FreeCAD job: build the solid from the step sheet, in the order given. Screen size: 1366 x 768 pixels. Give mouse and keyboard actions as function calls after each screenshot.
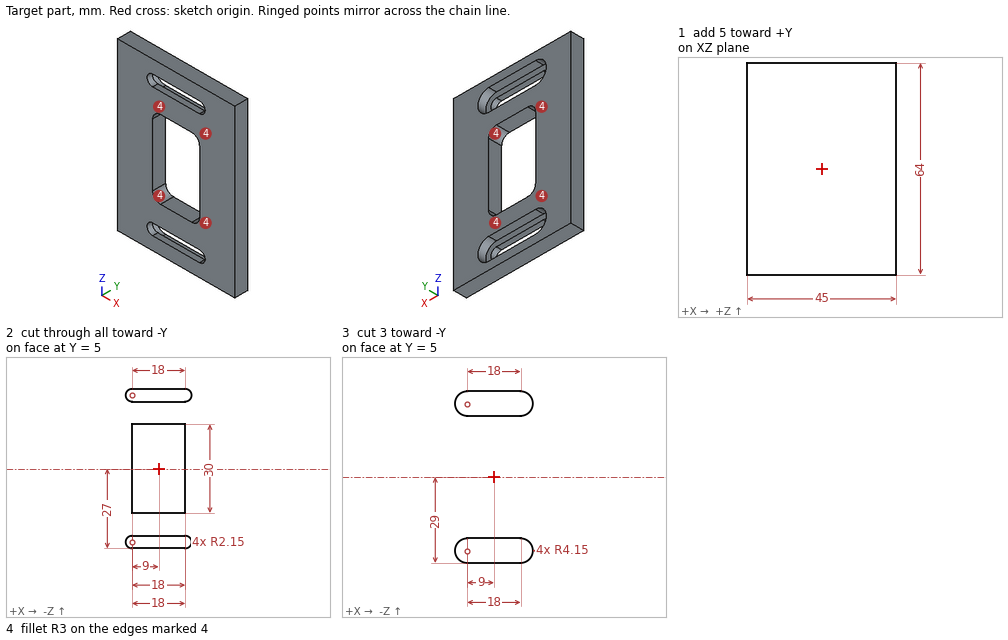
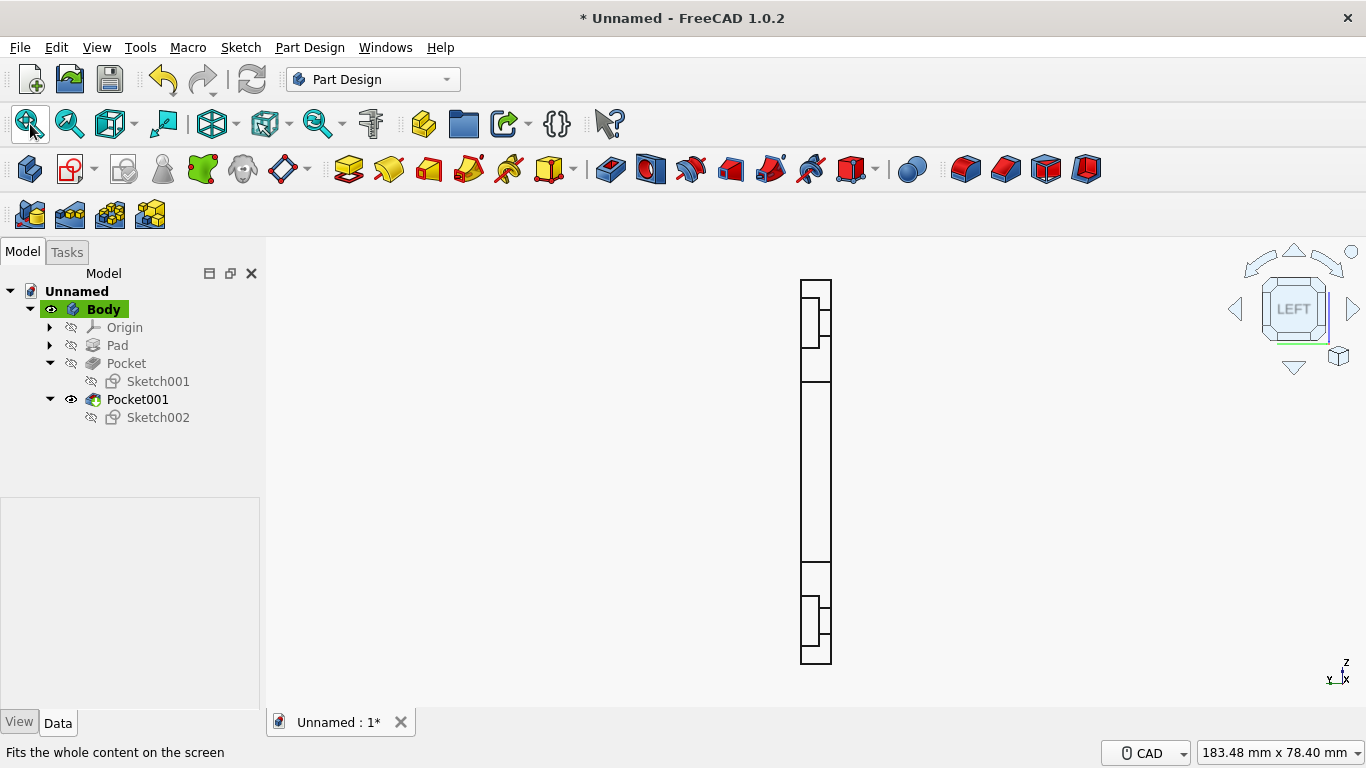
key(0)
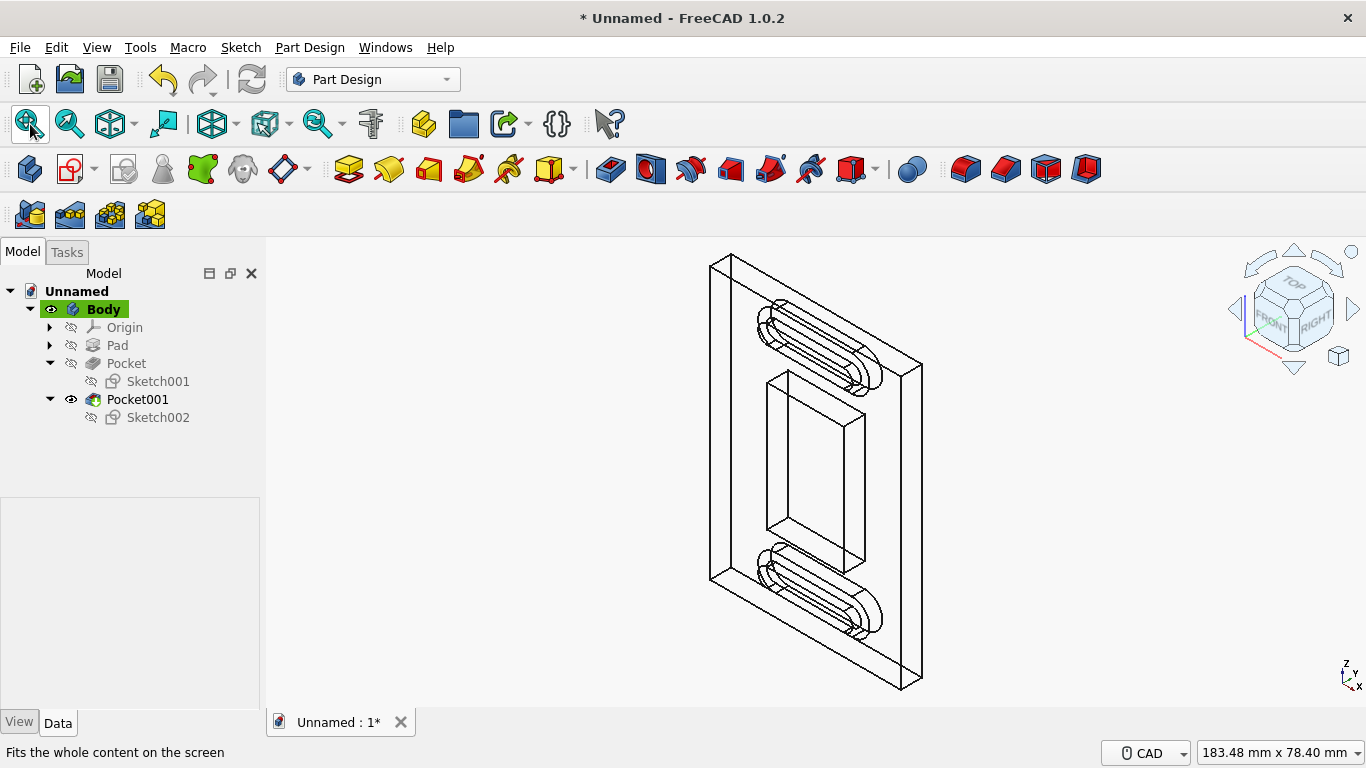
click(778, 522)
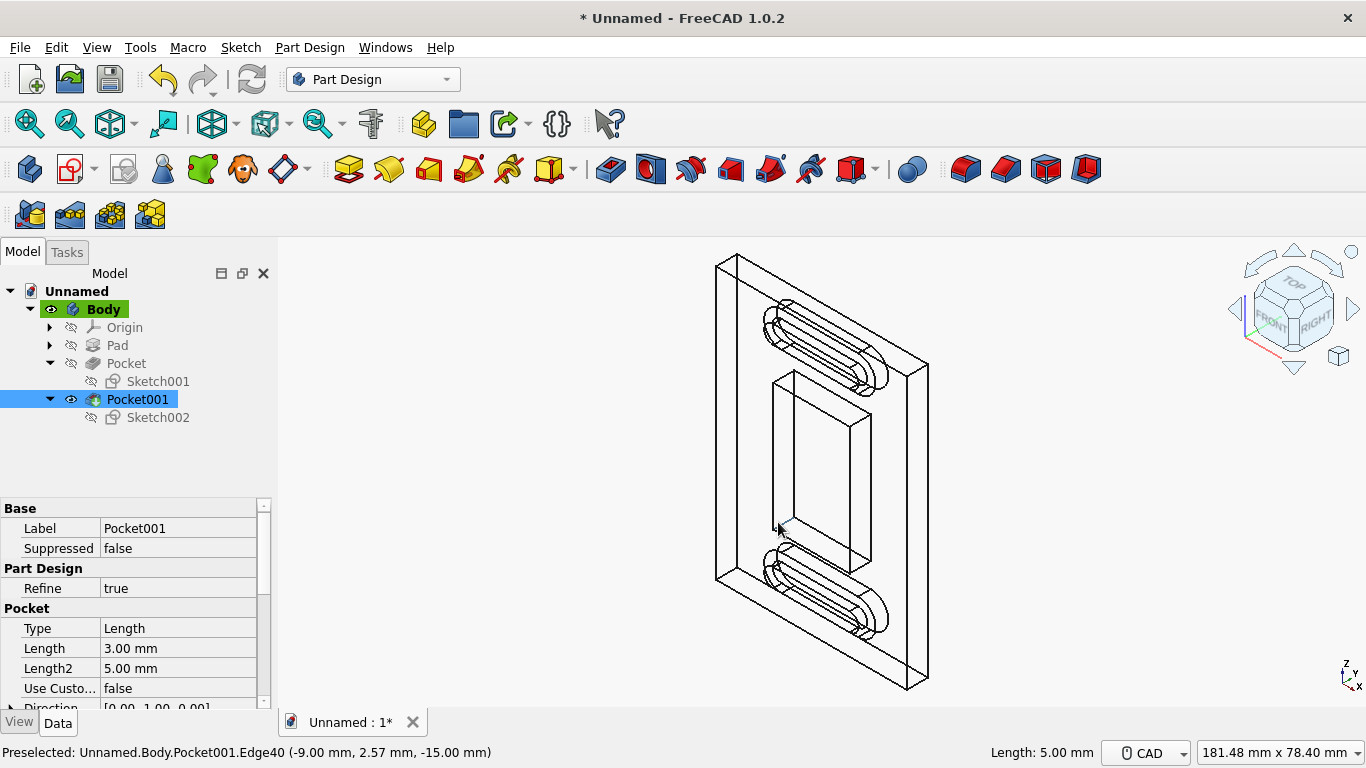
click(860, 566, ctrl)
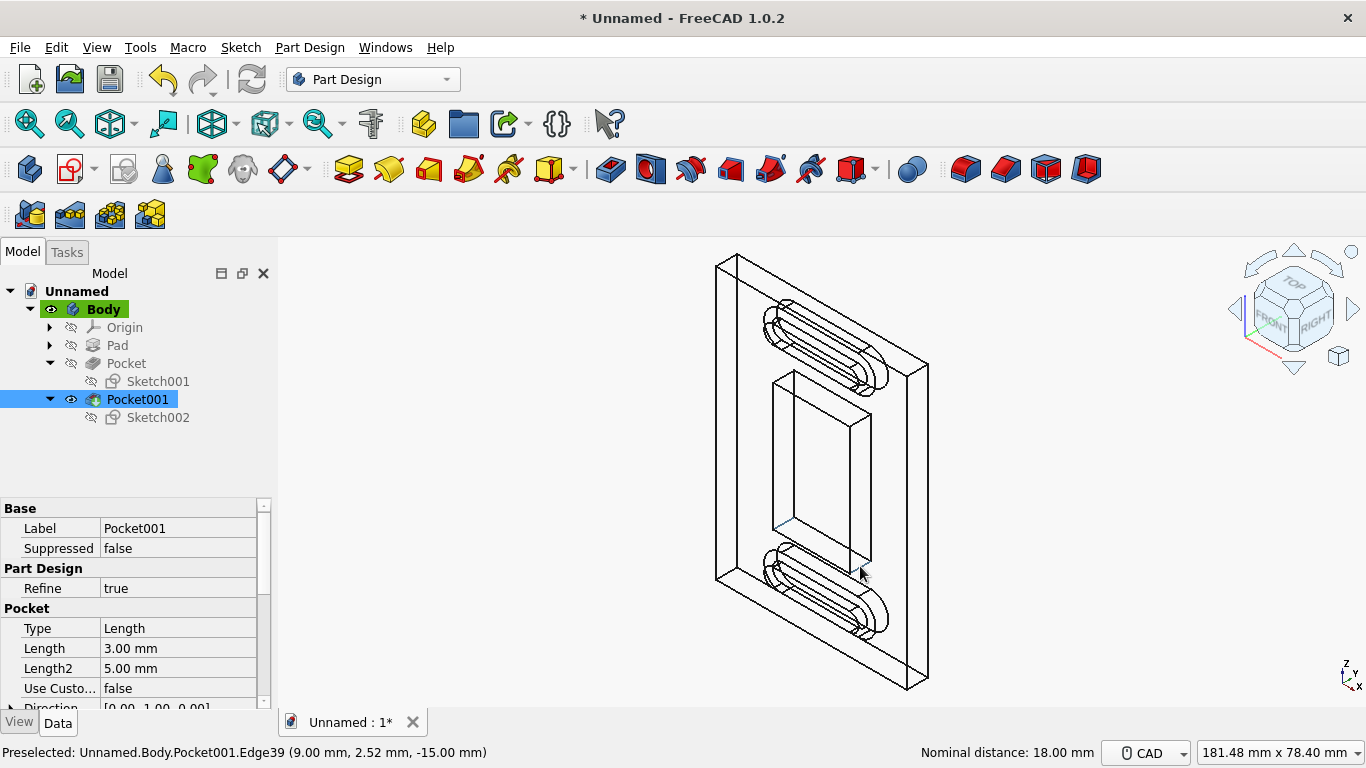
click(860, 420, ctrl)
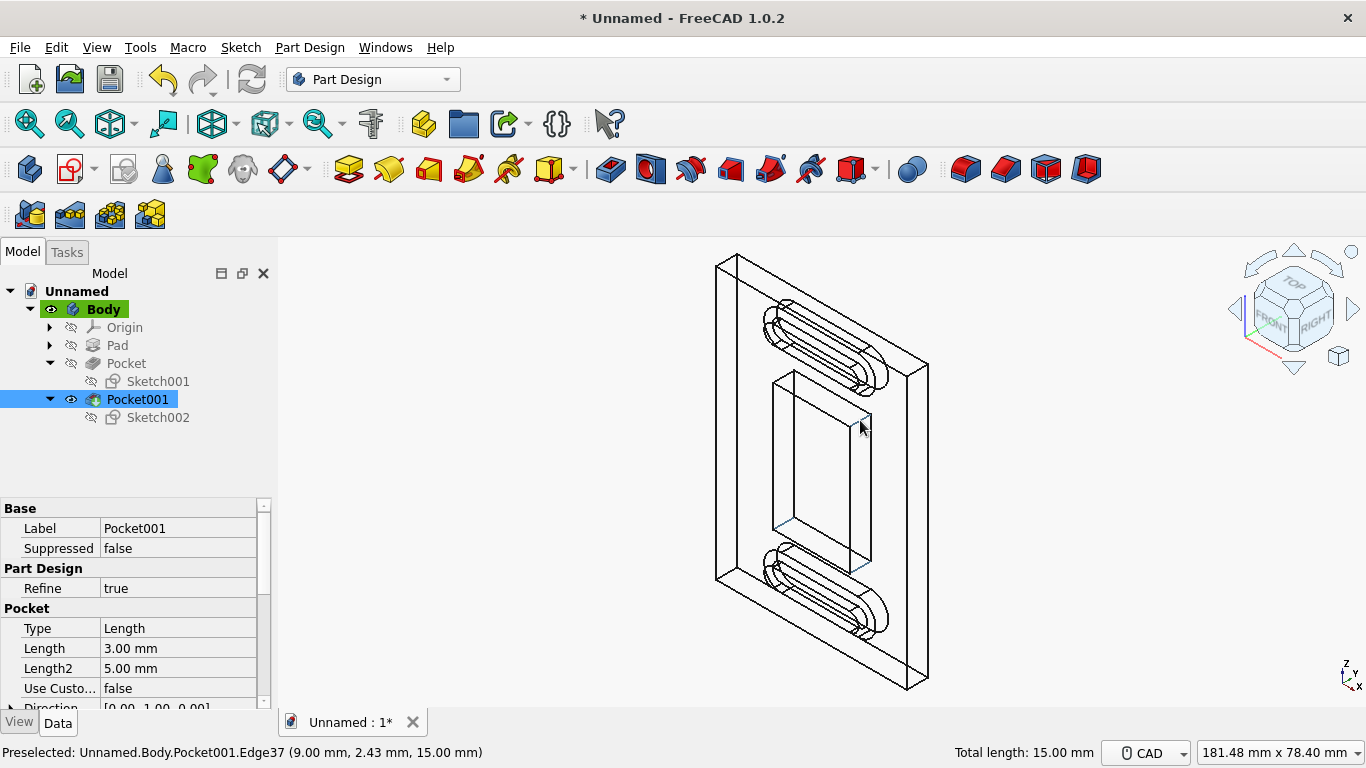
click(784, 376, ctrl)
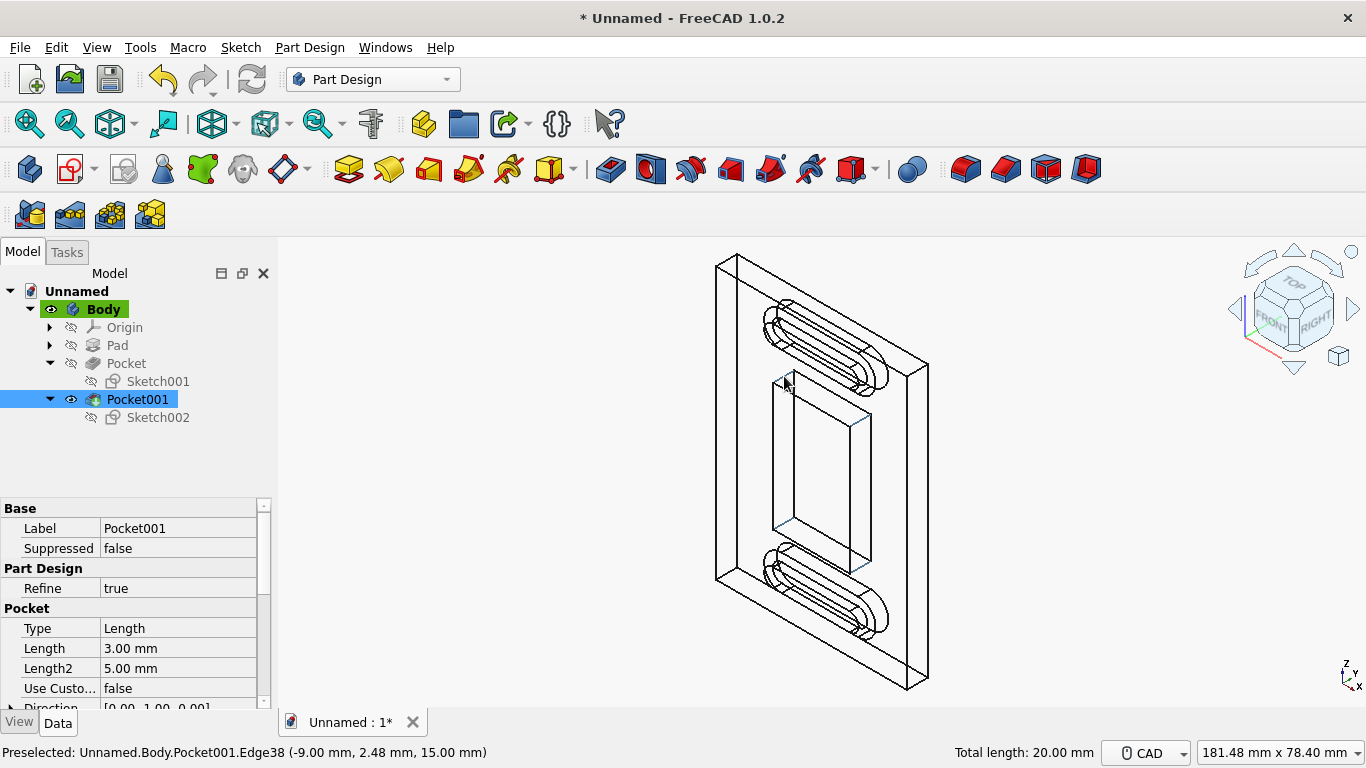
key(v)
key(1)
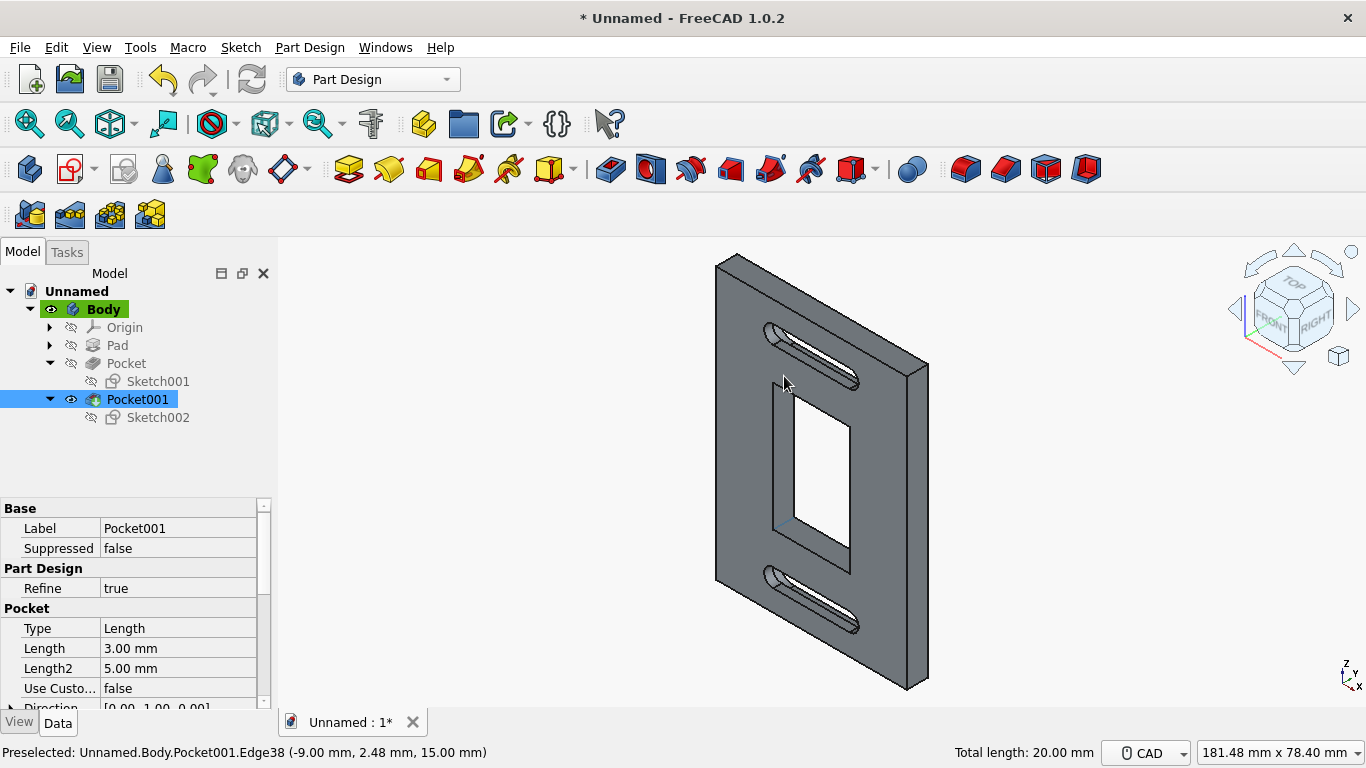
click(966, 170)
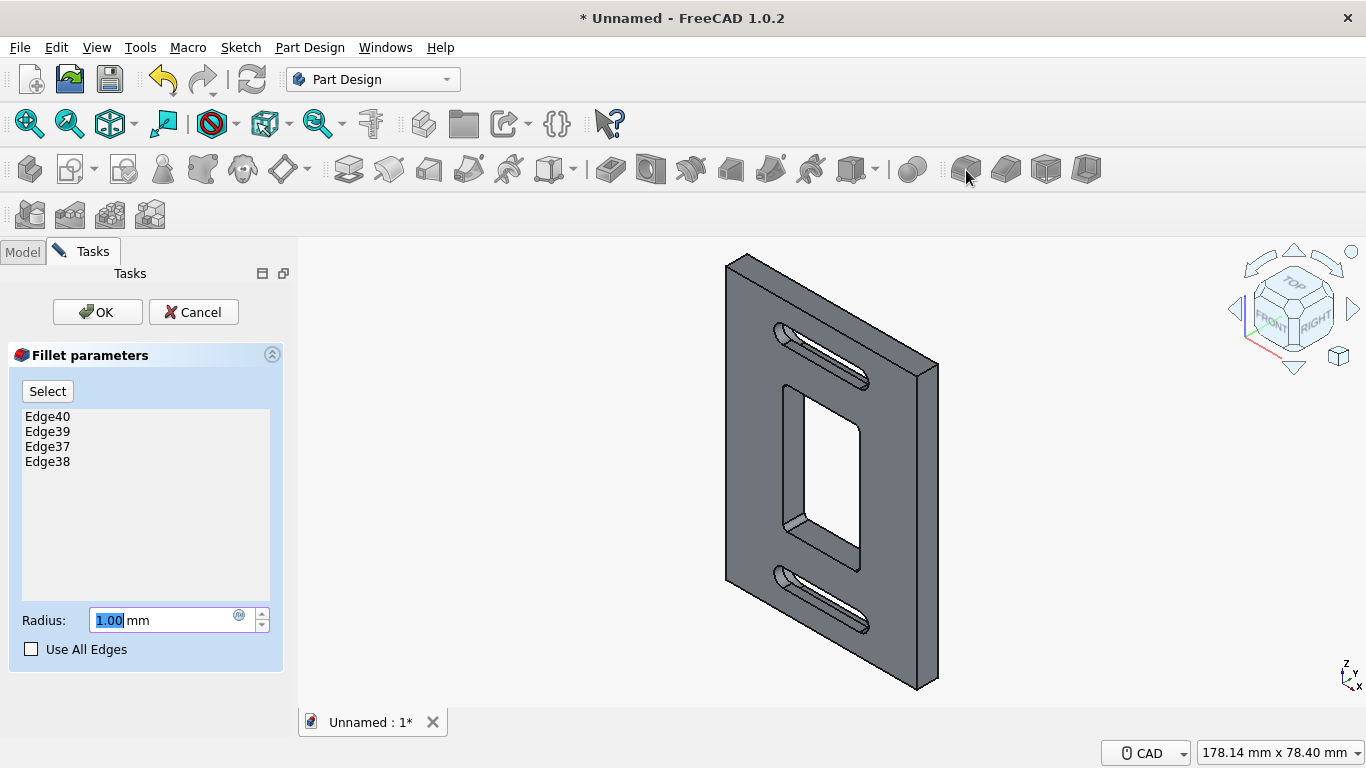
text(3)
key(Tab)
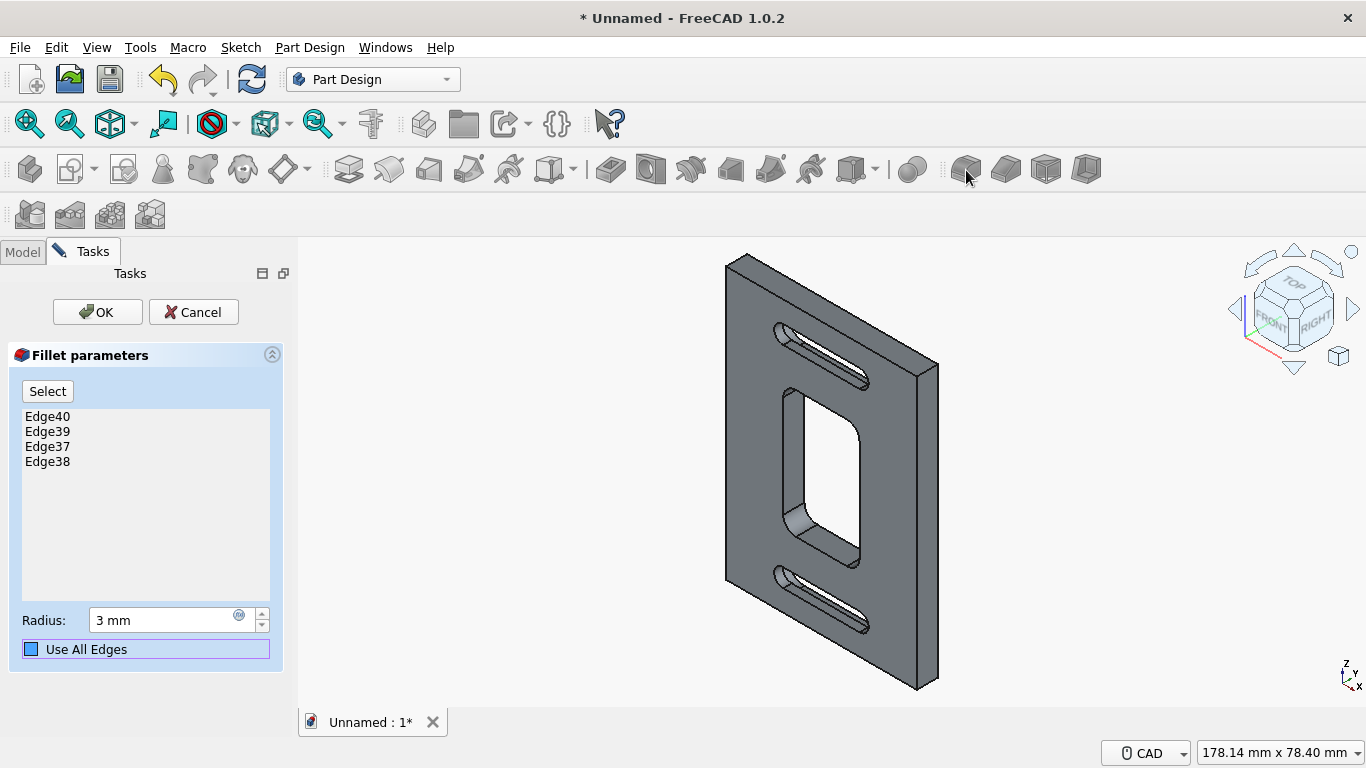
click(98, 312)